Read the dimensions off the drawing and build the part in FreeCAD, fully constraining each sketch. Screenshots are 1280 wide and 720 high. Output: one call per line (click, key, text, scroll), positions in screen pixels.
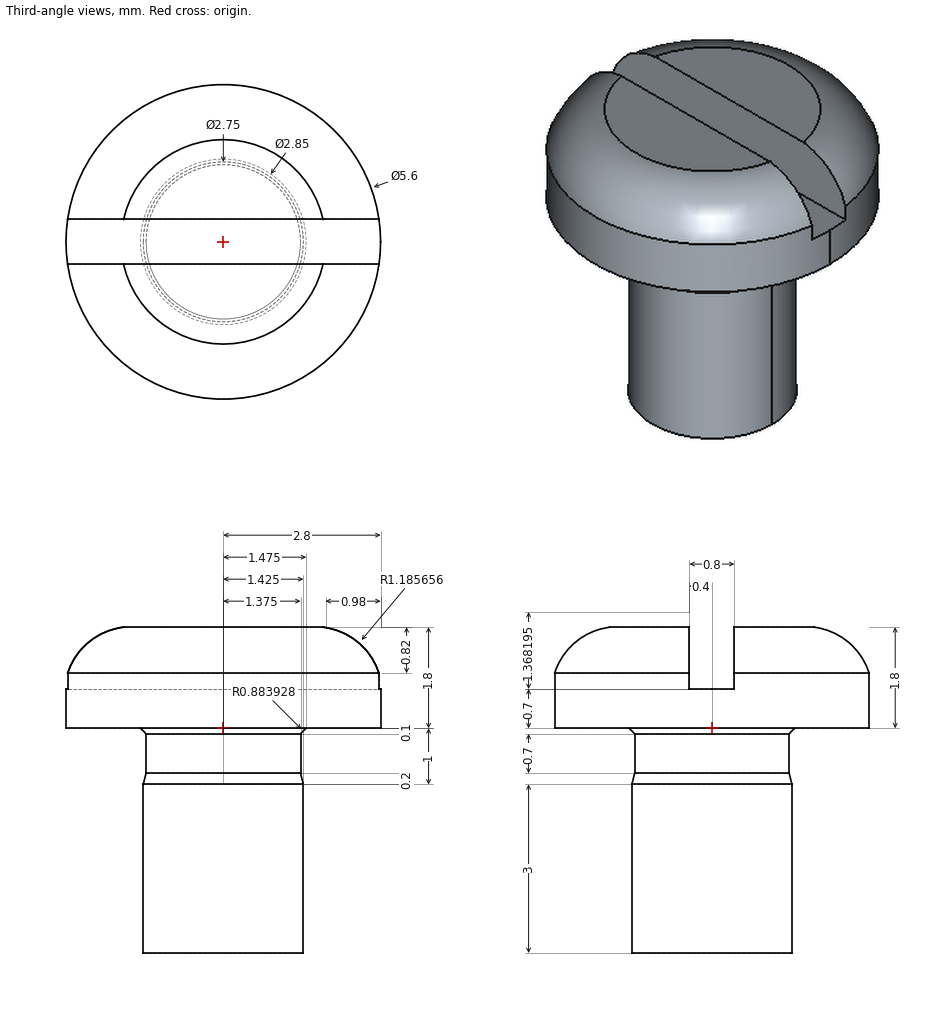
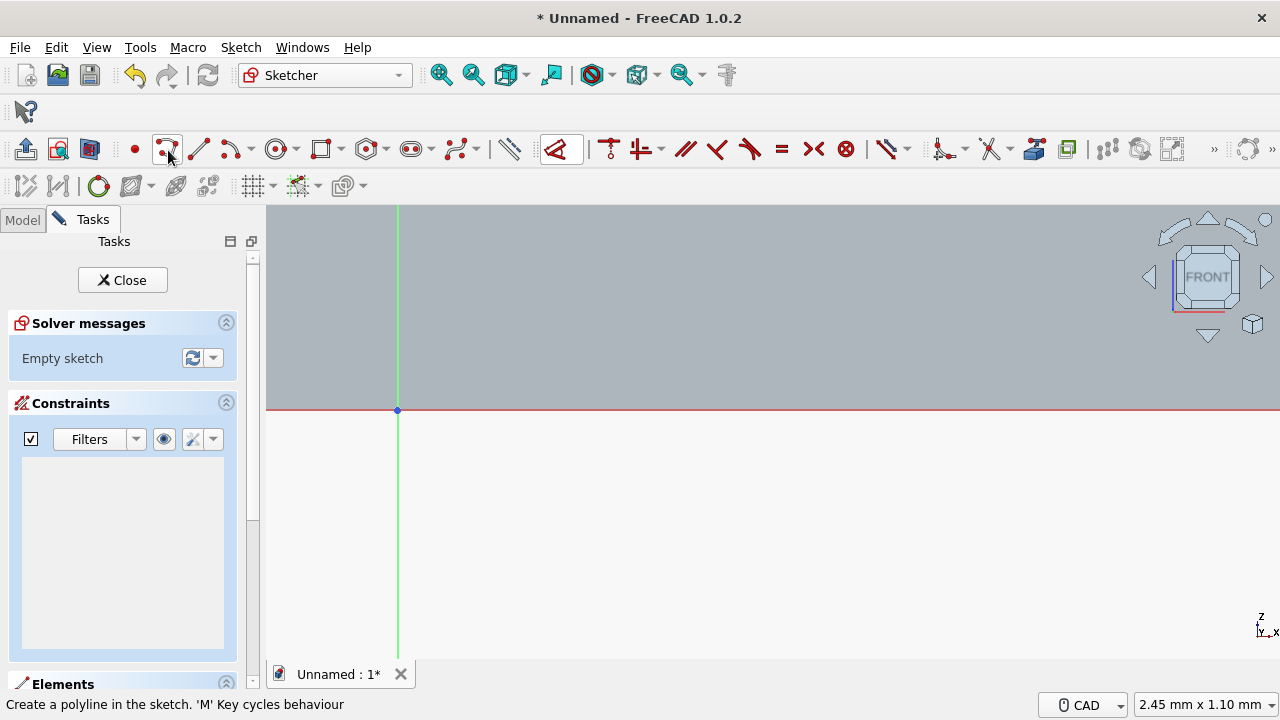
click(966, 451)
click(398, 451)
click(398, 410)
click(1008, 419)
right_click(1008, 419)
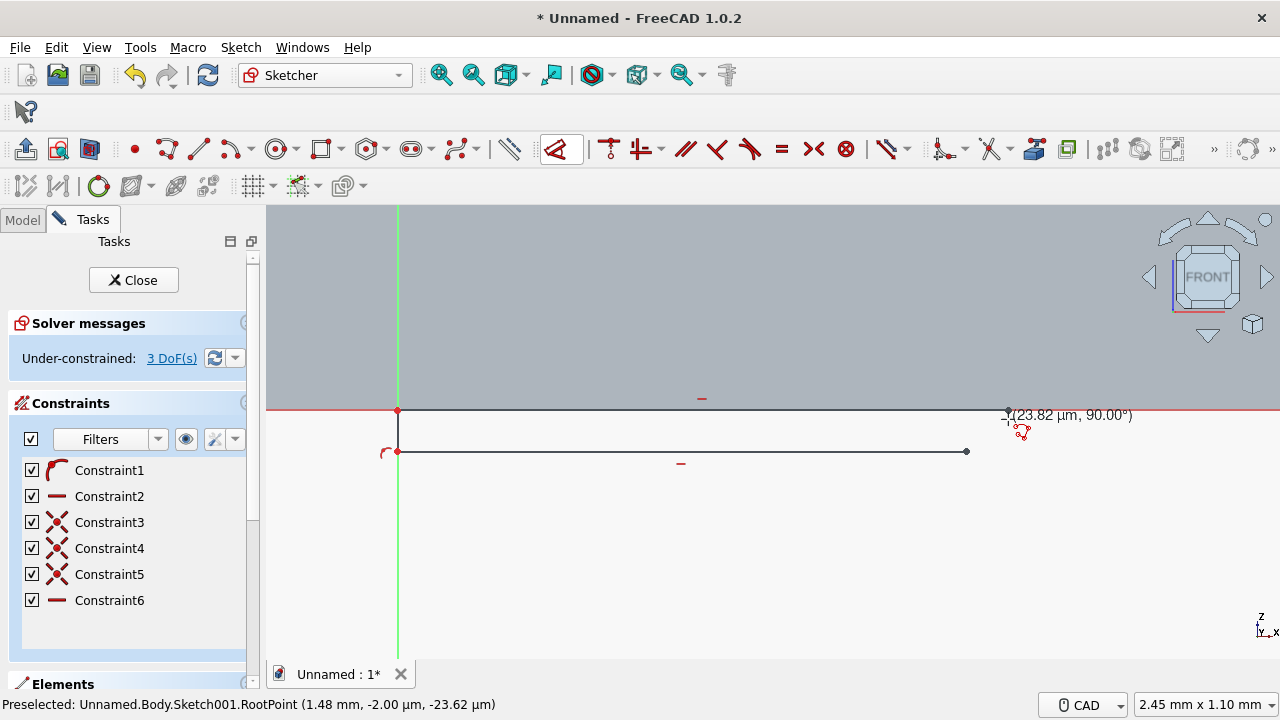
click(254, 150)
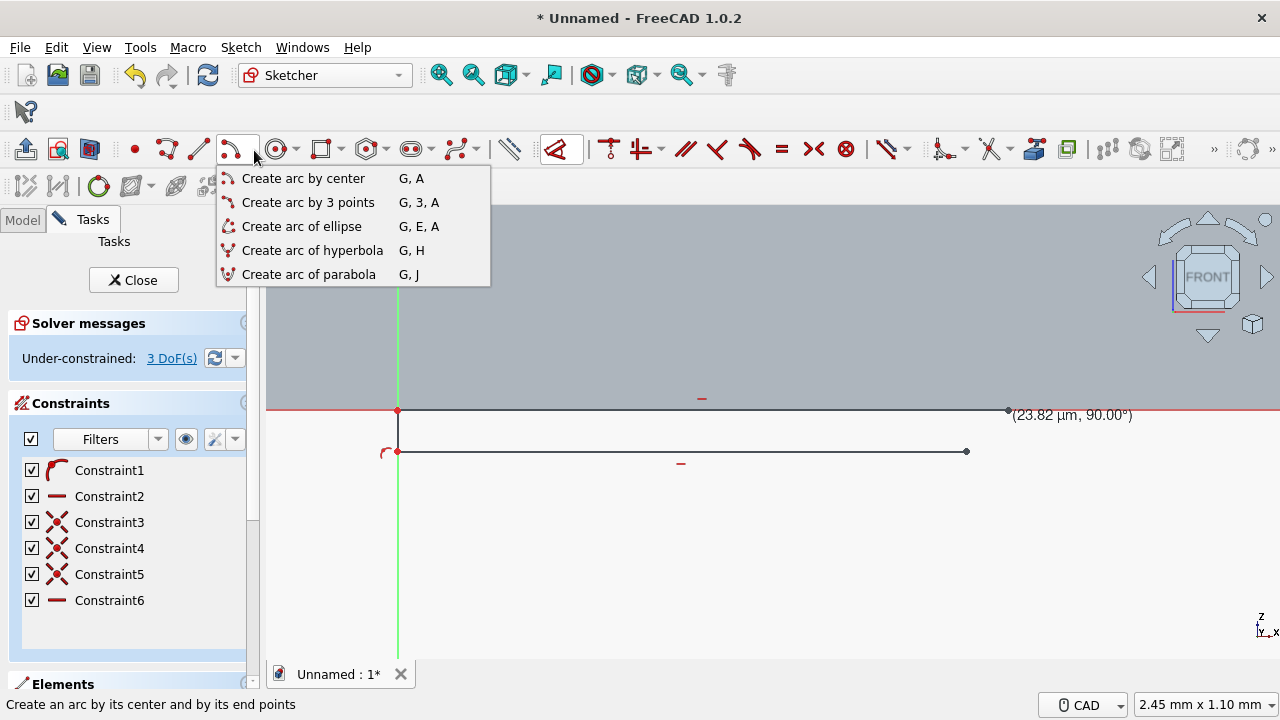
click(354, 202)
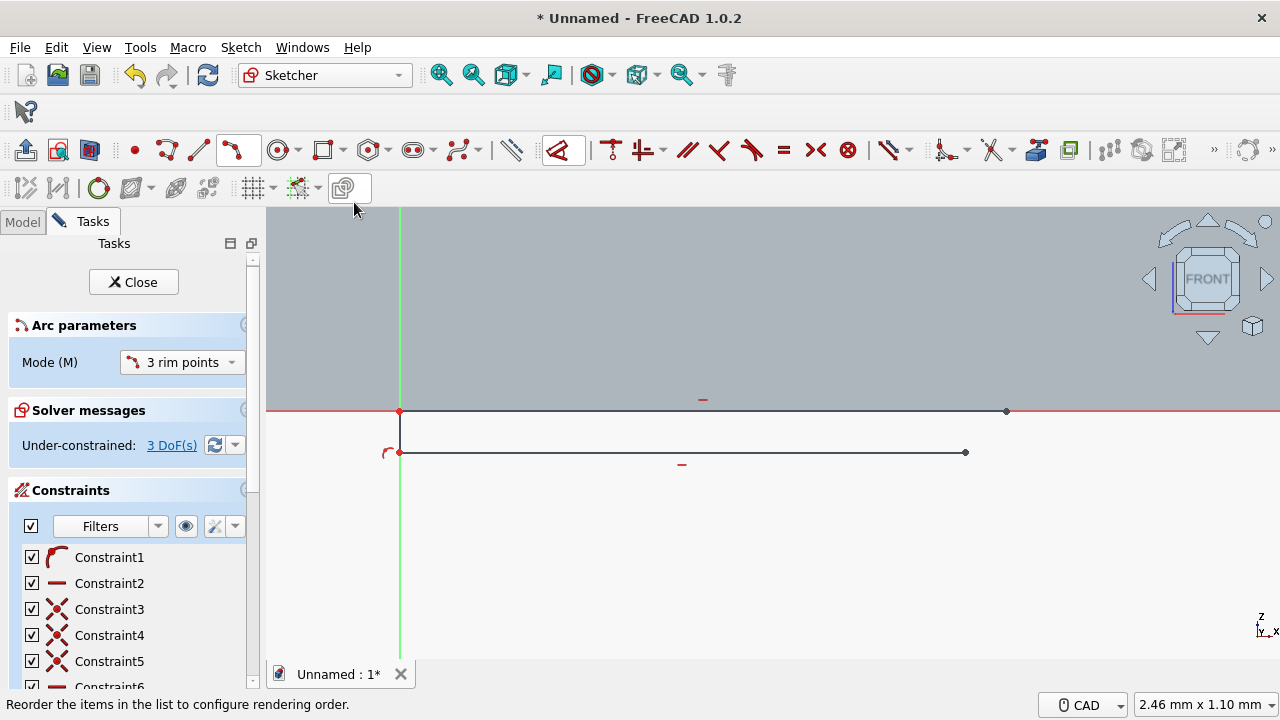
click(1007, 411)
click(965, 453)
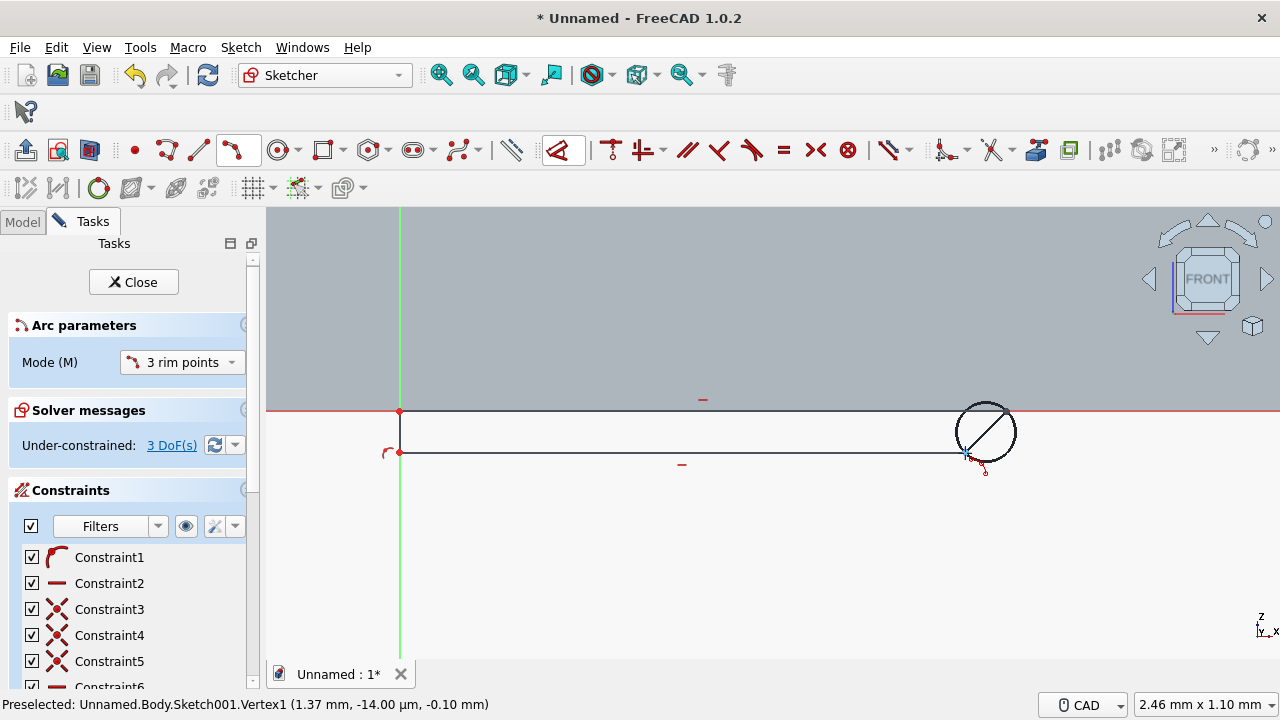
scroll(985, 431, up, 14)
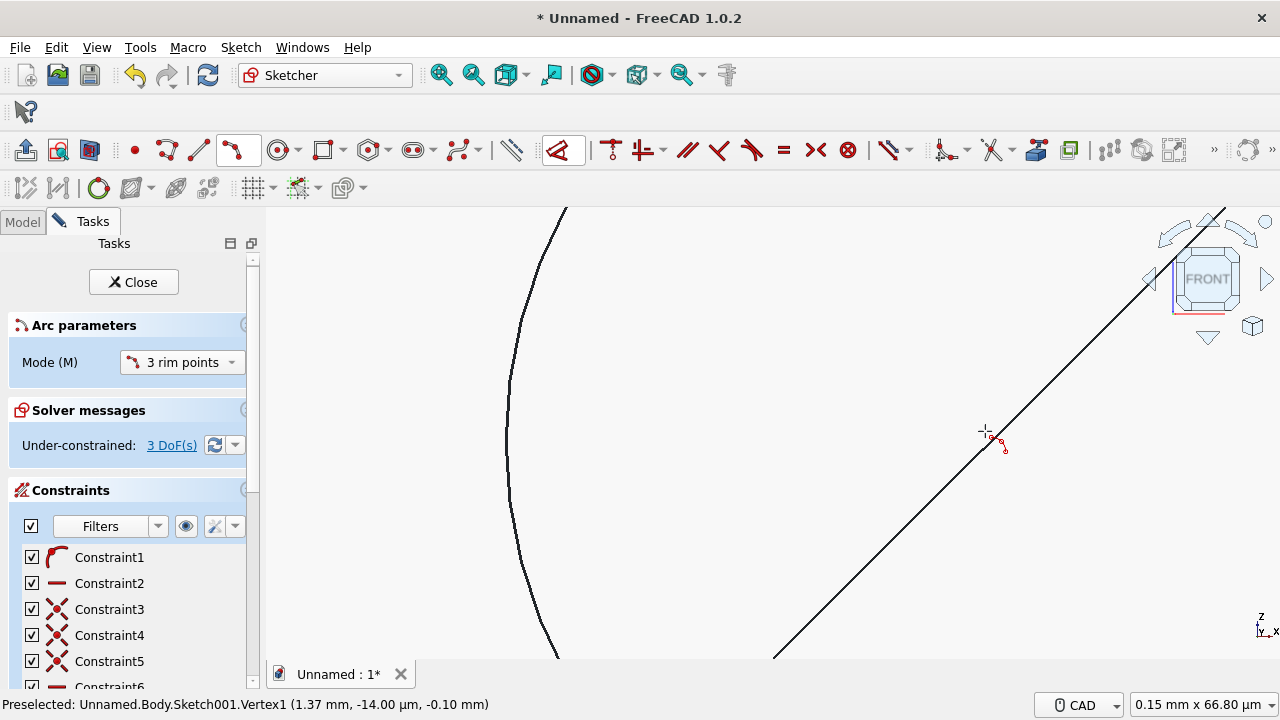
click(976, 423)
key(Escape)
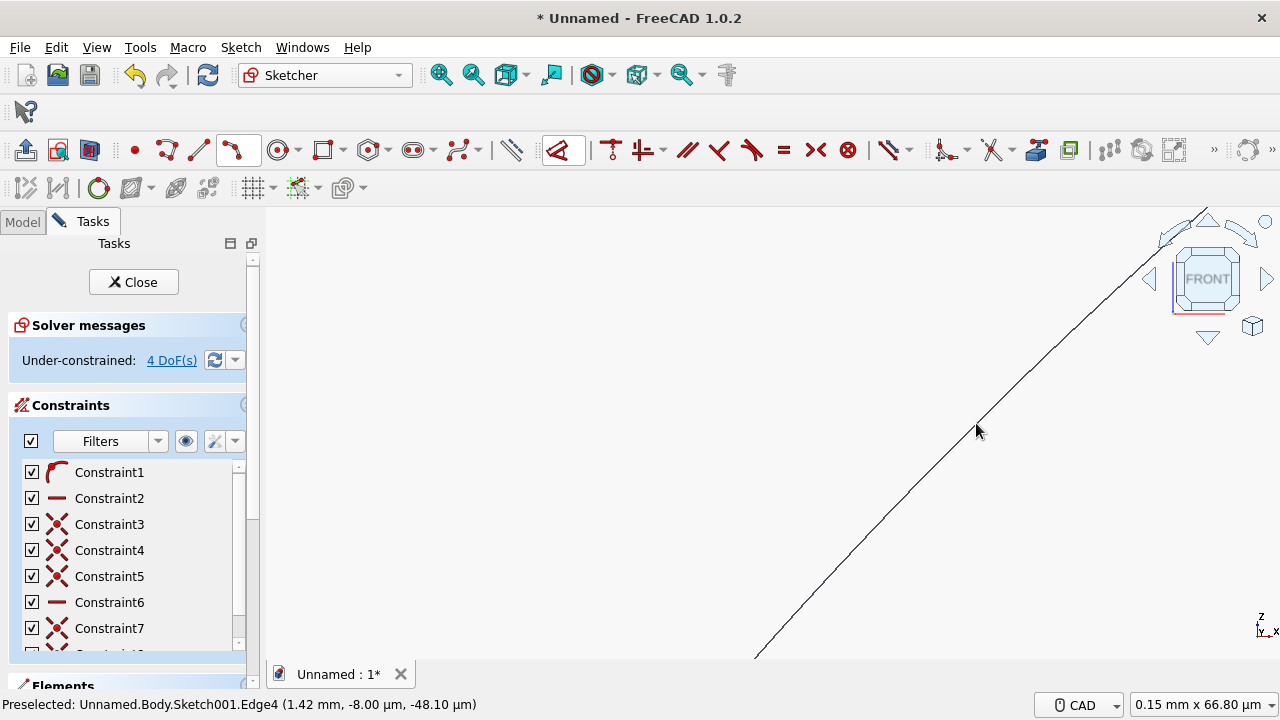
scroll(987, 433, down, 14)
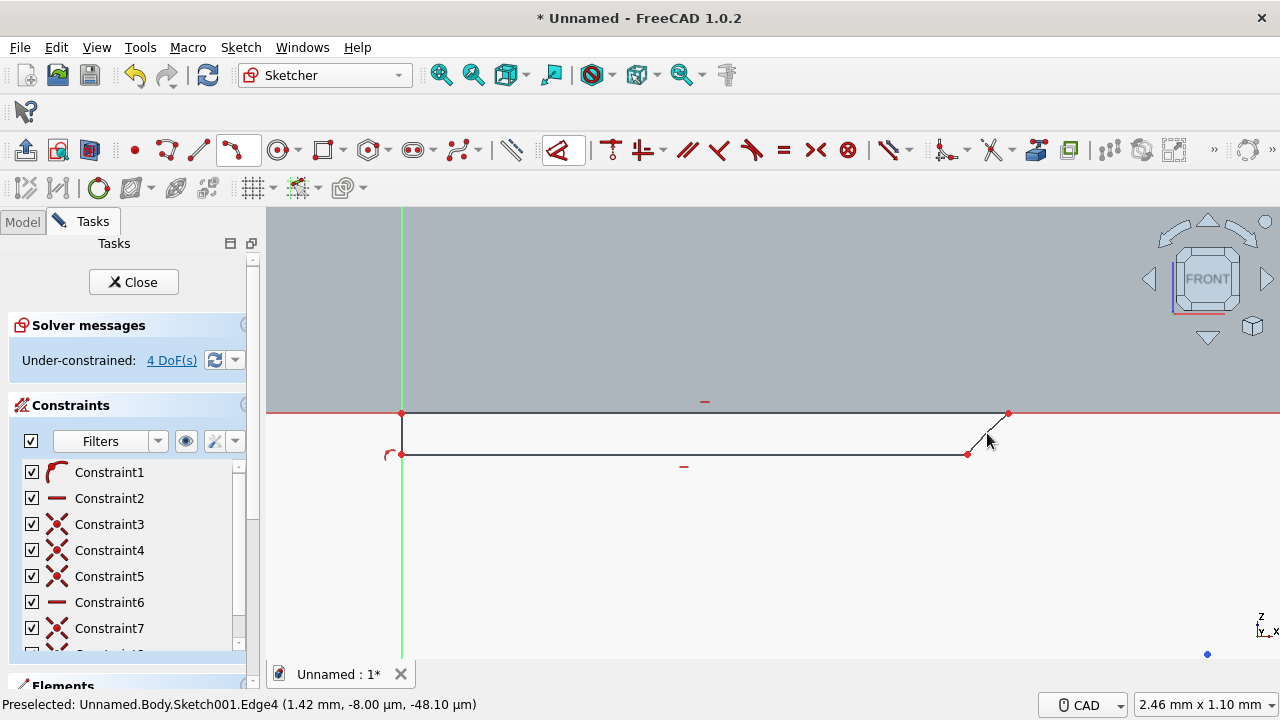
click(979, 441)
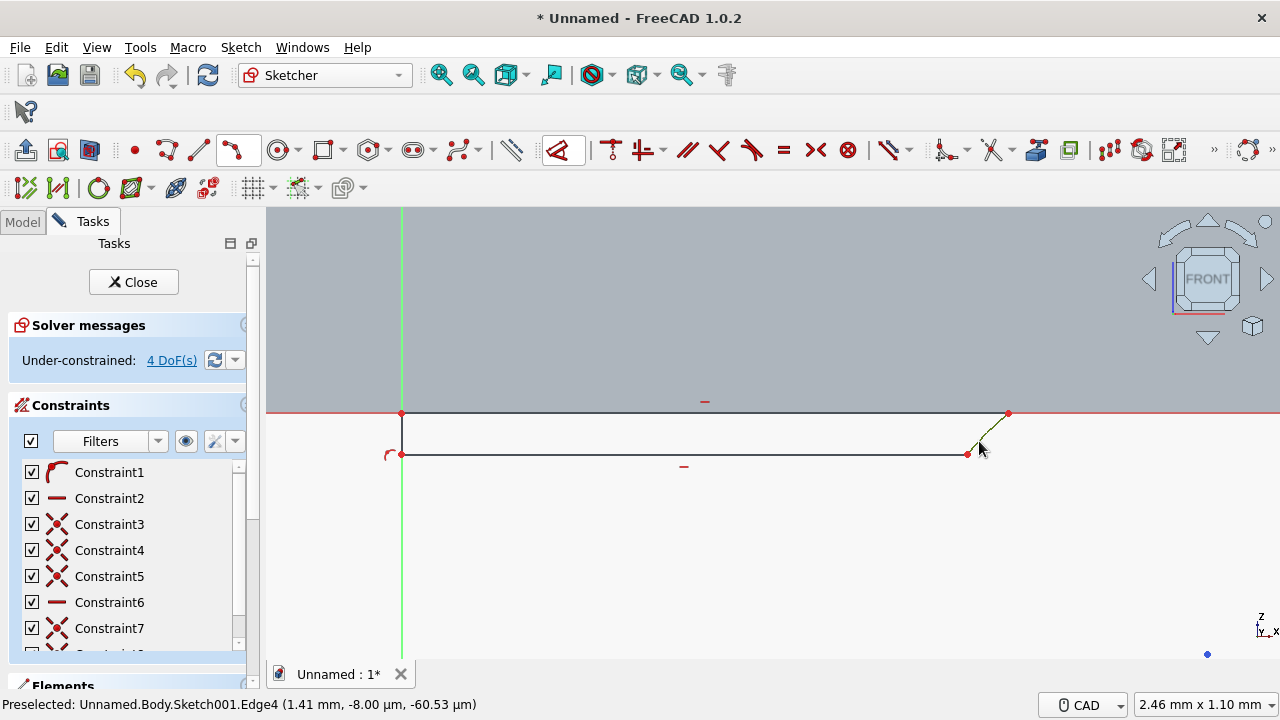
key(k)
key(r)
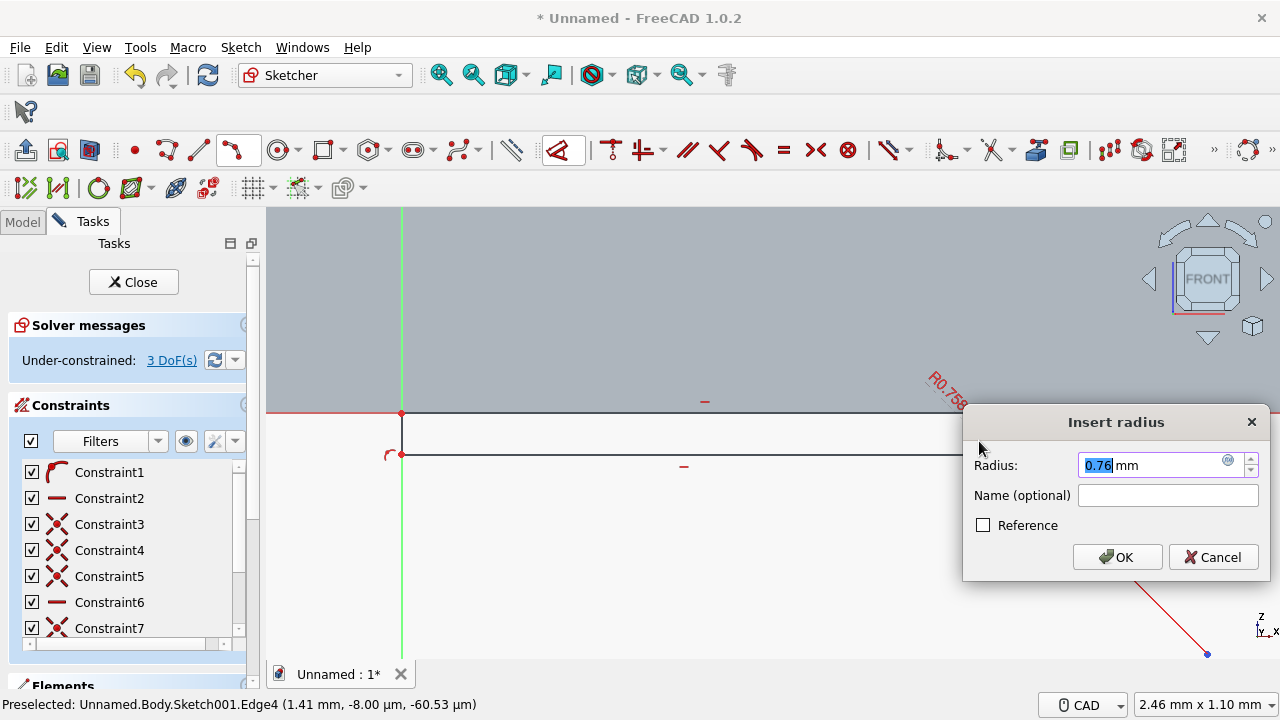
text(0.883928)
key(Return)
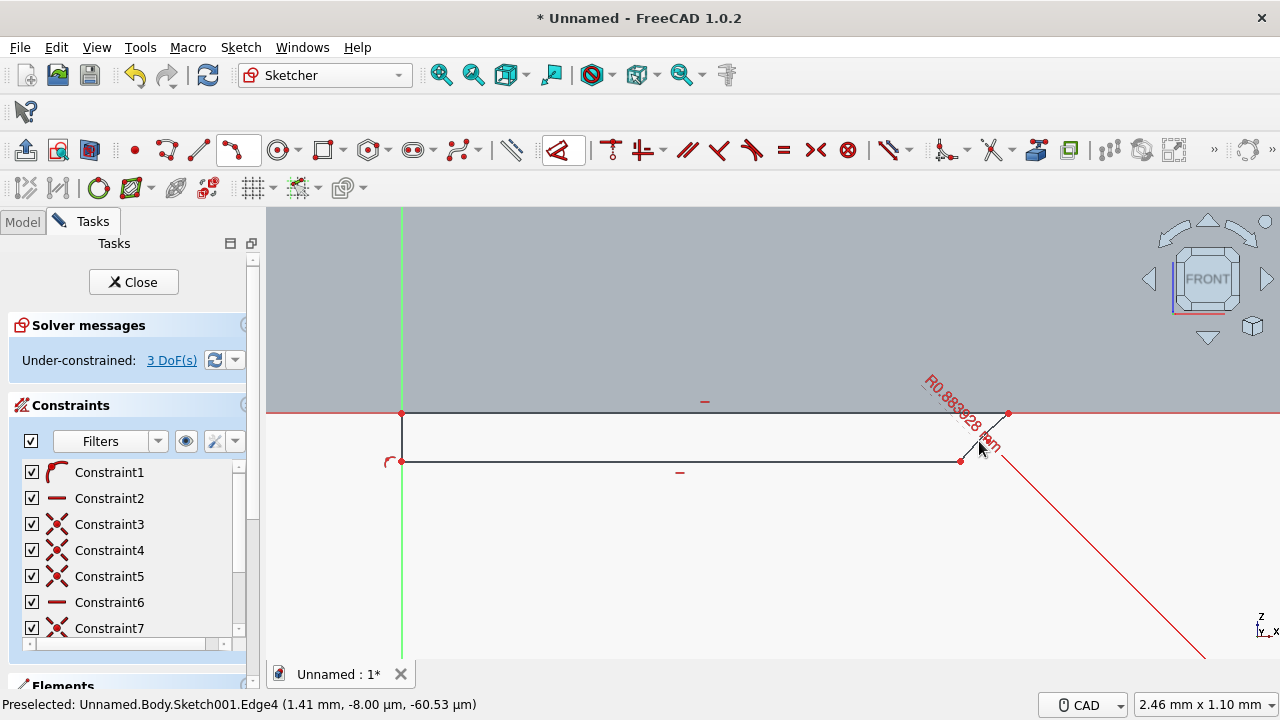
click(402, 447)